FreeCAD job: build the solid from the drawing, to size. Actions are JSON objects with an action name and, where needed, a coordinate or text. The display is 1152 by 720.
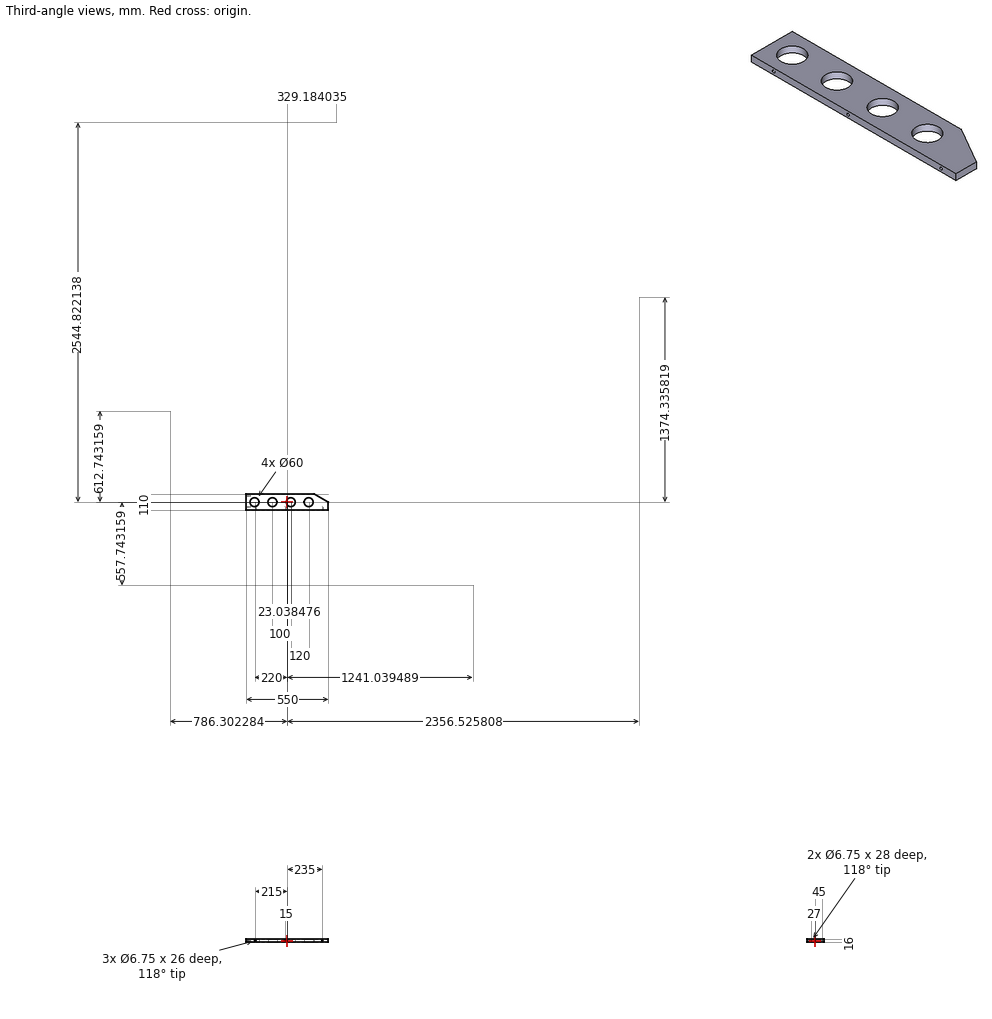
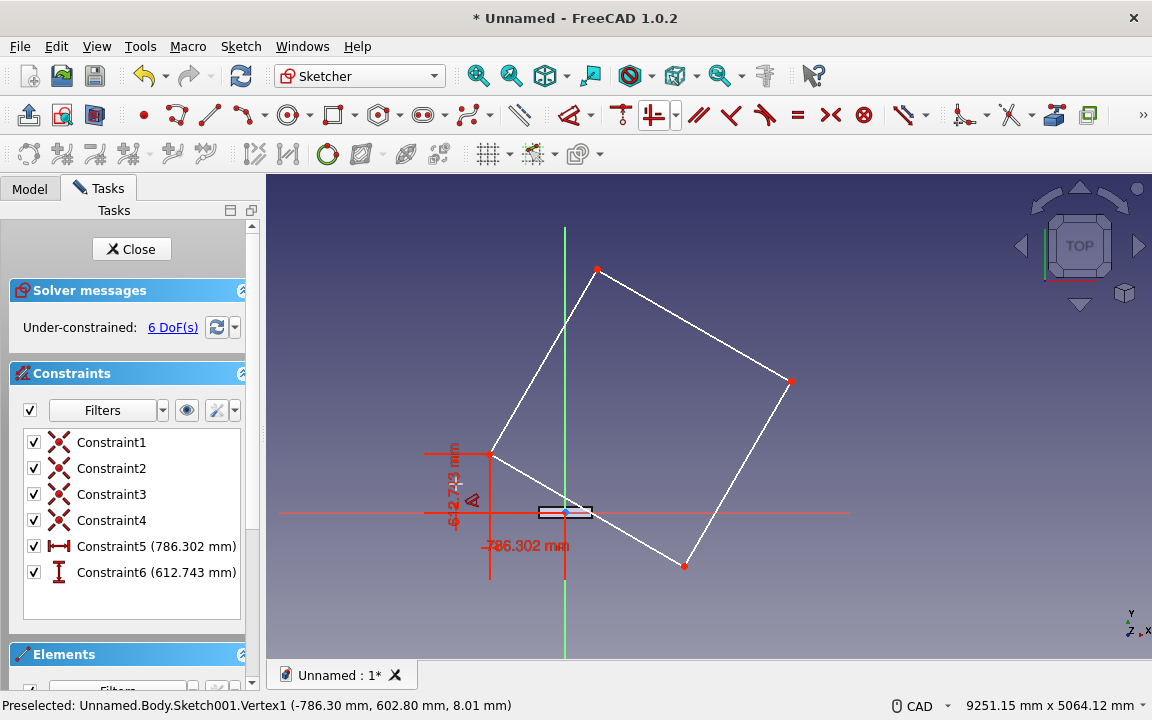
{"action": "left_click", "coordinate": [684, 567]}
{"action": "left_click", "coordinate": [718, 540]}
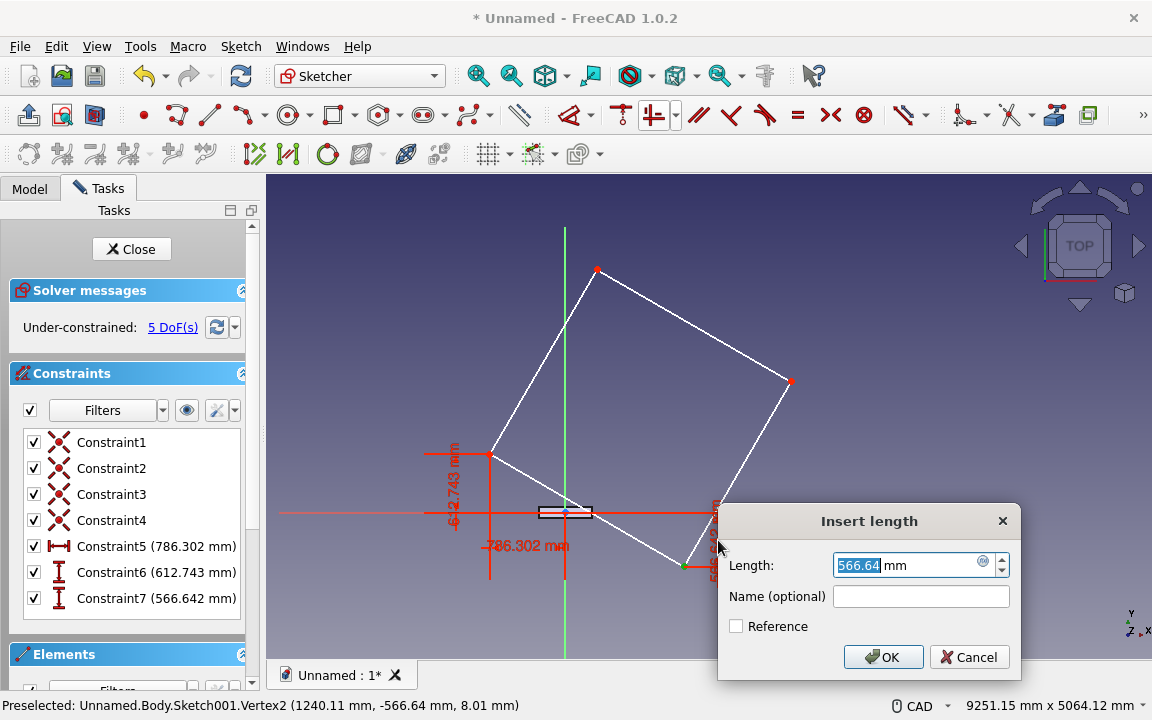
{"action": "type", "text": "557.743159"}
{"action": "key", "text": "Return"}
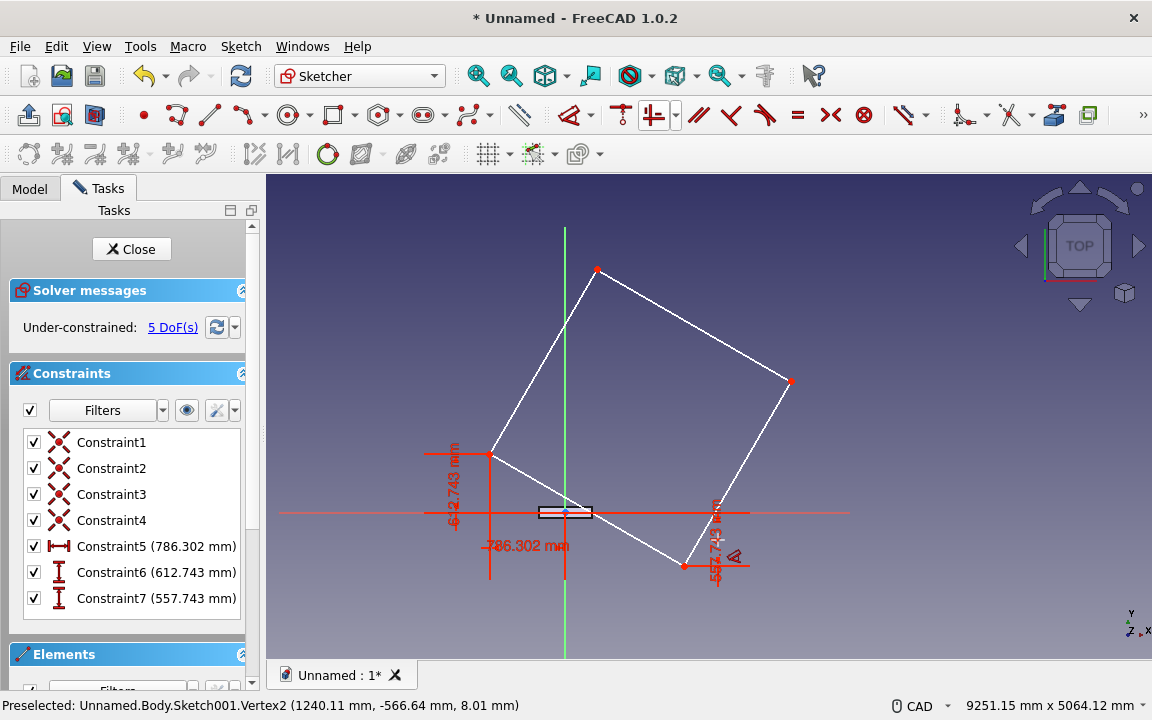
{"action": "scroll", "coordinate": [597, 270], "scroll_direction": "up", "scroll_amount": 2}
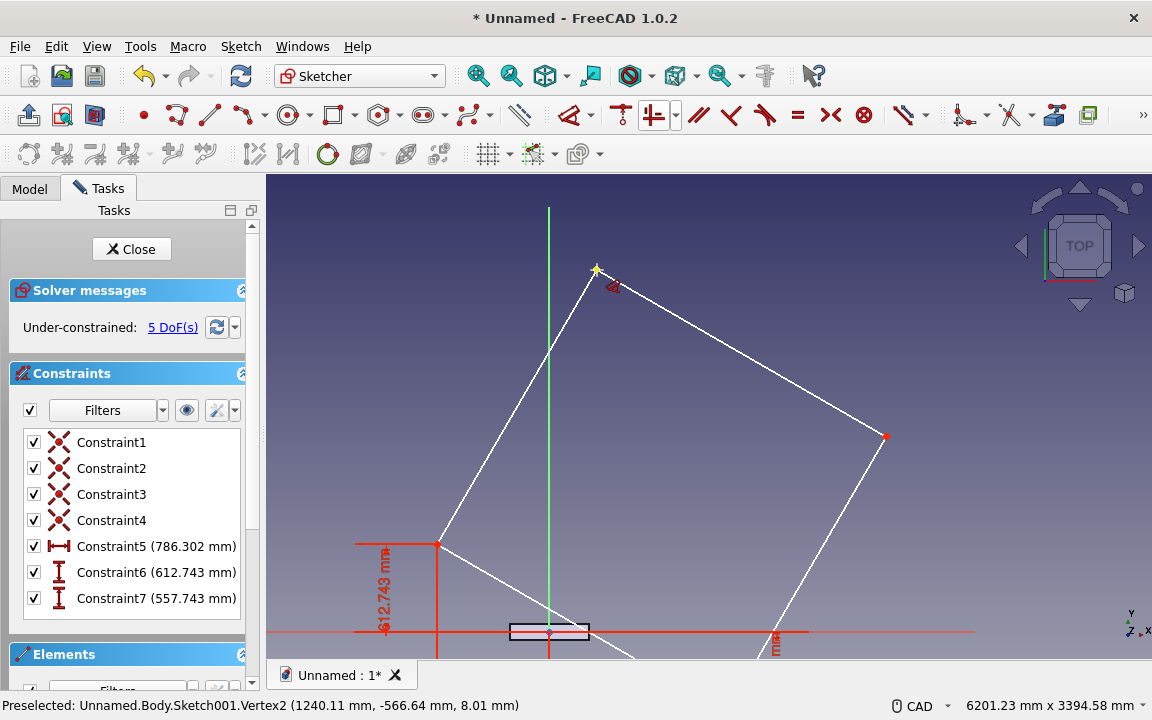
{"action": "left_click", "coordinate": [597, 270]}
{"action": "left_click", "coordinate": [573, 236]}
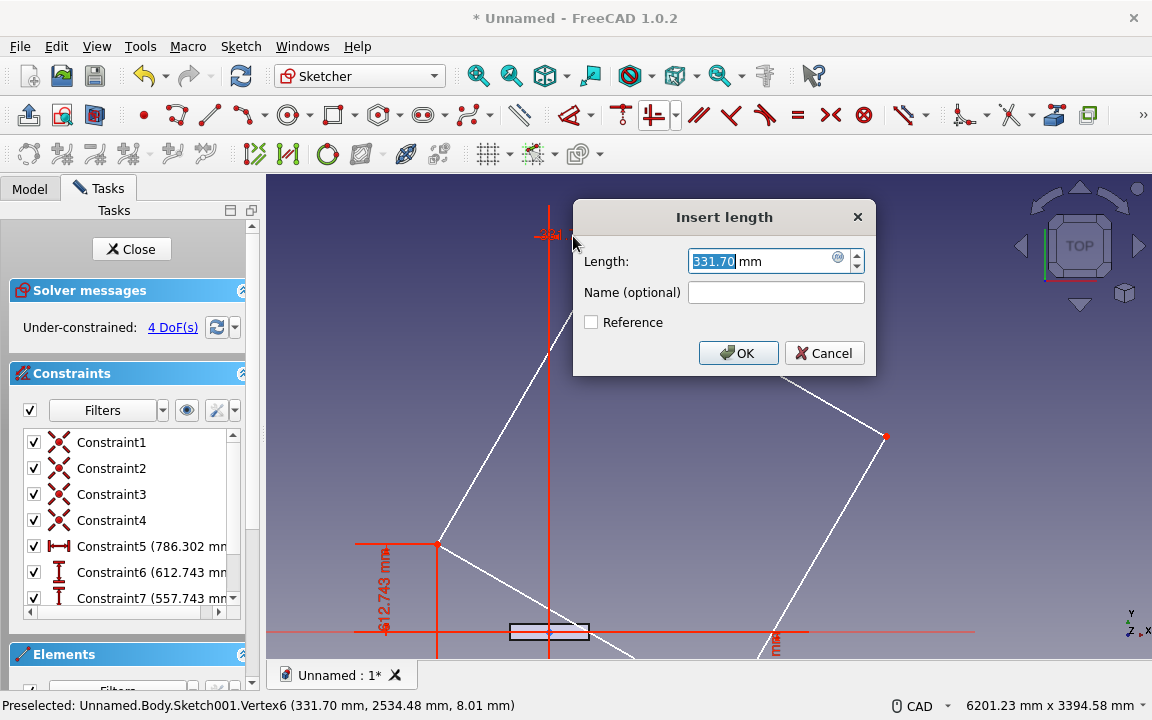
{"action": "type", "text": "329.184035"}
{"action": "key", "text": "Return"}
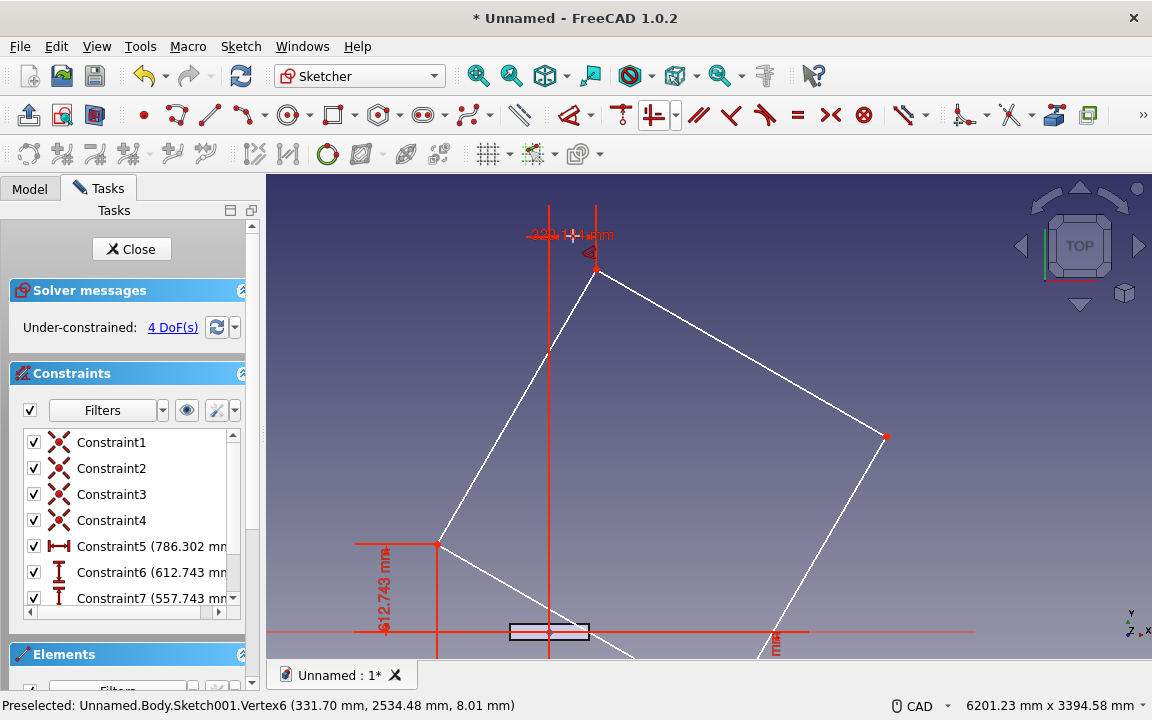
{"action": "scroll", "coordinate": [598, 267], "scroll_direction": "down", "scroll_amount": 2}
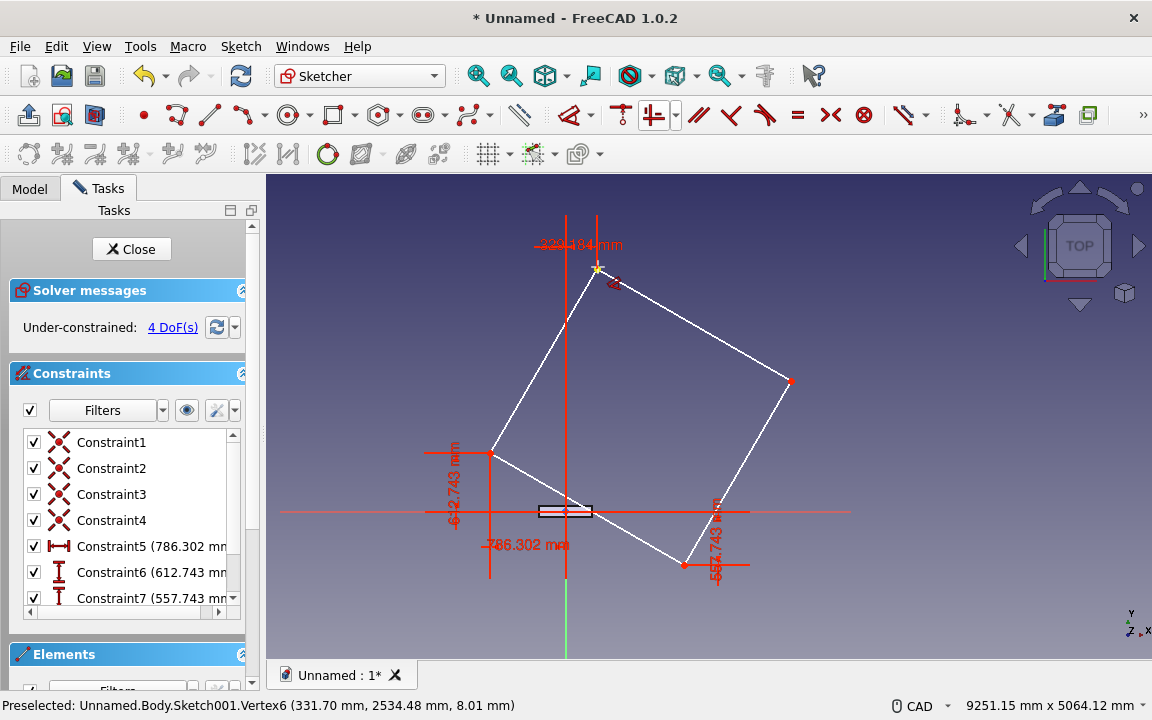
{"action": "left_click", "coordinate": [684, 565]}
{"action": "left_click", "coordinate": [625, 599]}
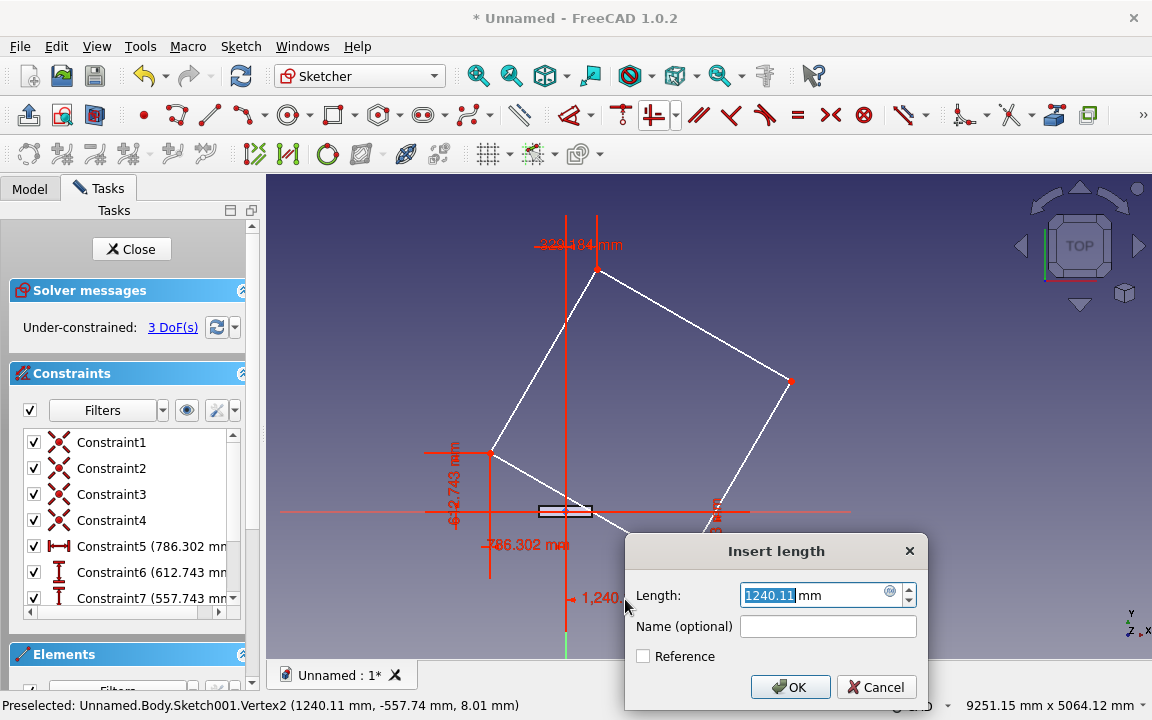
{"action": "type", "text": "1241.039489"}
{"action": "key", "text": "Return"}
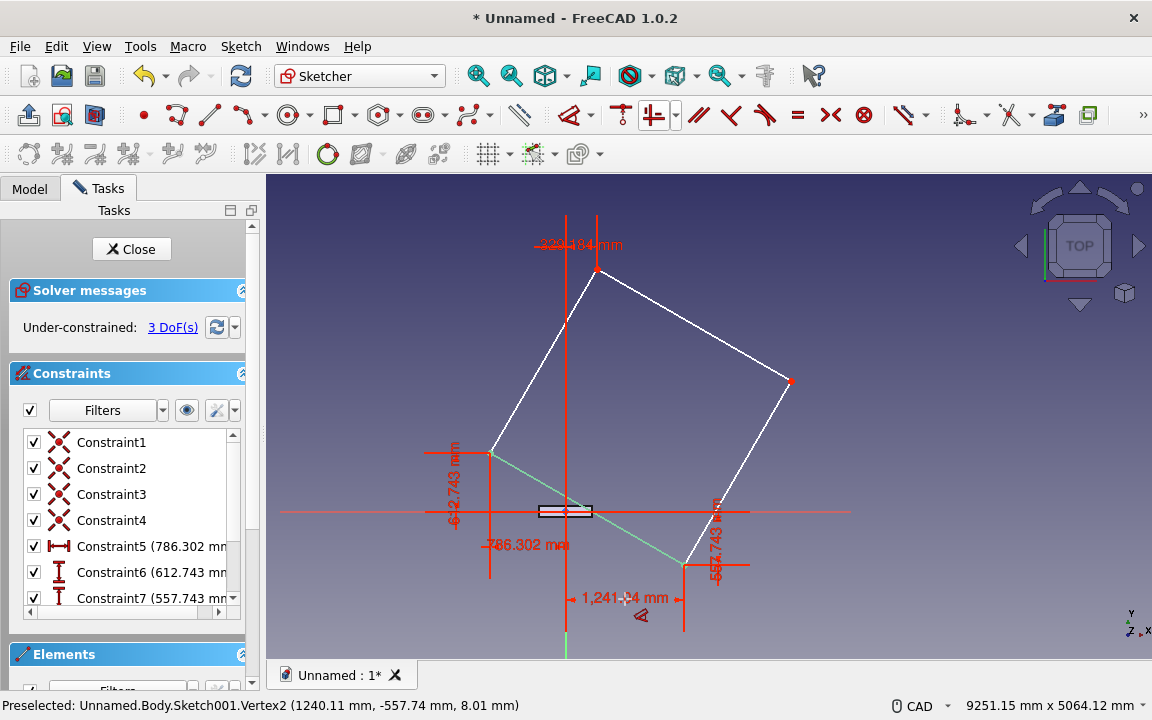
{"action": "left_click", "coordinate": [791, 381]}
{"action": "left_click", "coordinate": [599, 546]}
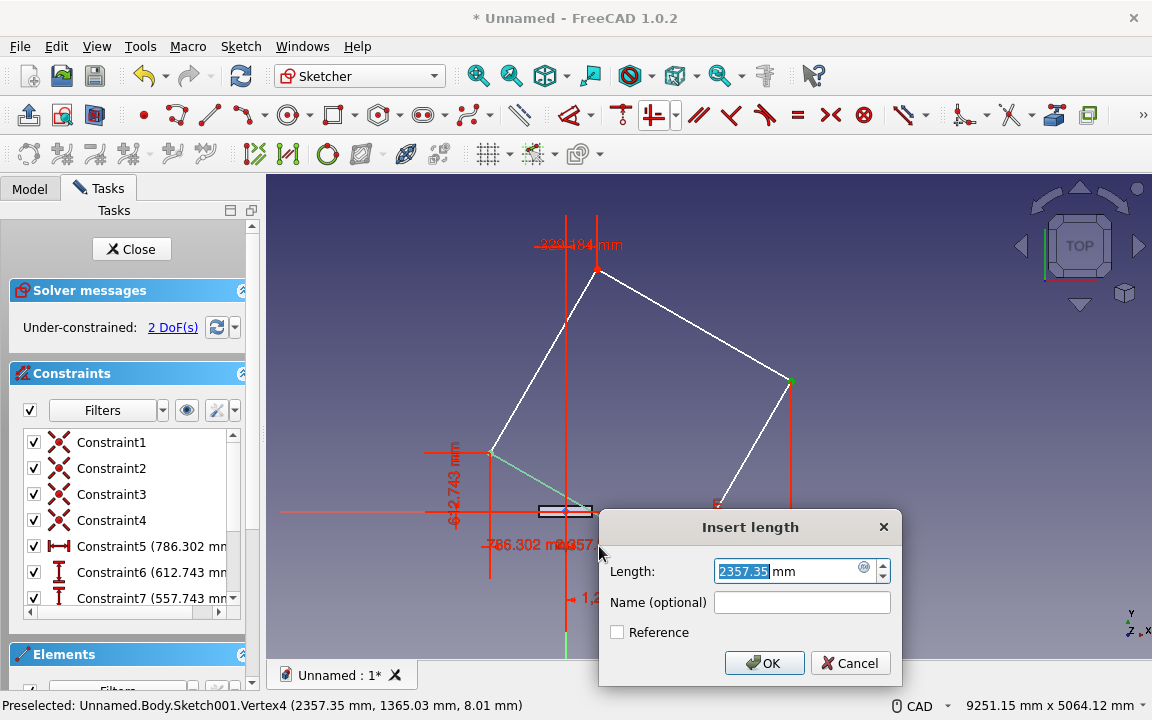
{"action": "type", "text": "2356.525808"}
{"action": "key", "text": "Return"}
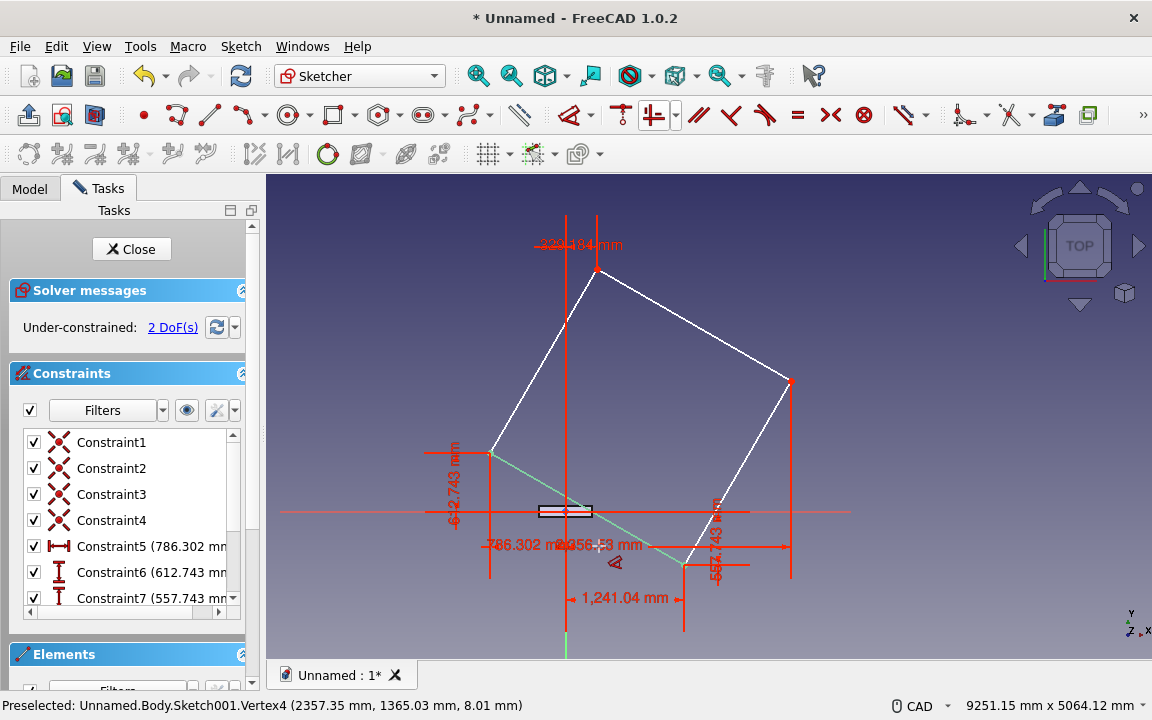
{"action": "left_click", "coordinate": [791, 381]}
{"action": "left_click", "coordinate": [825, 446]}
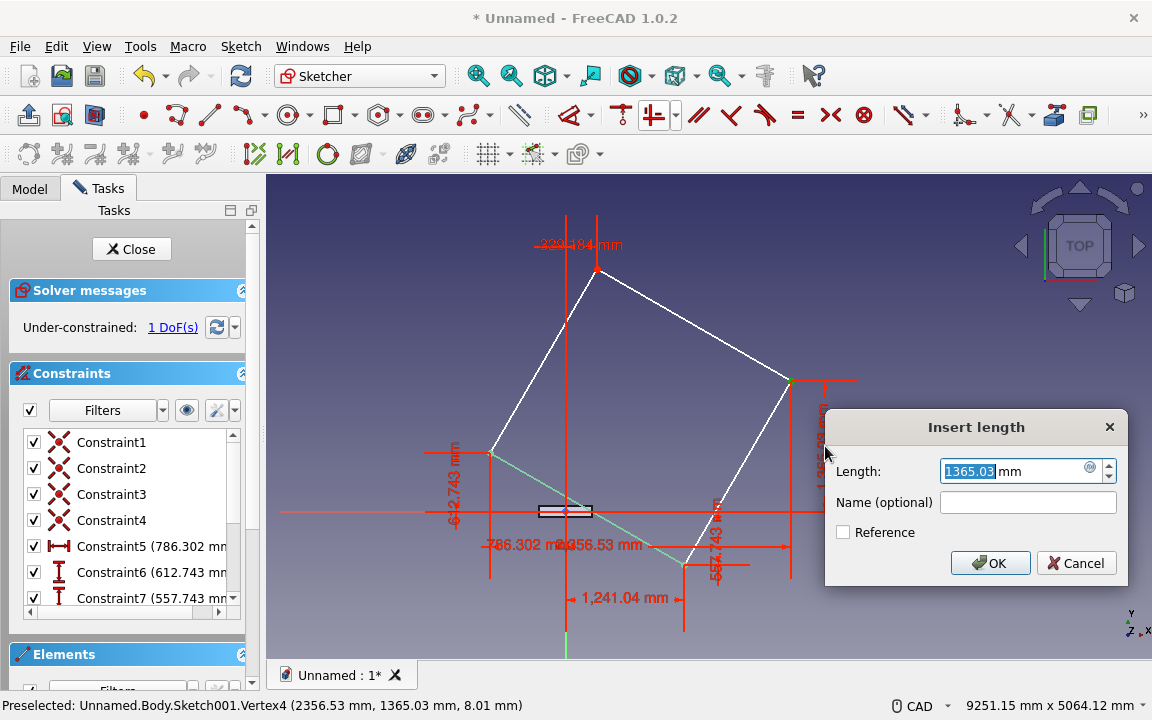
{"action": "type", "text": "1374.335819"}
{"action": "key", "text": "Return"}